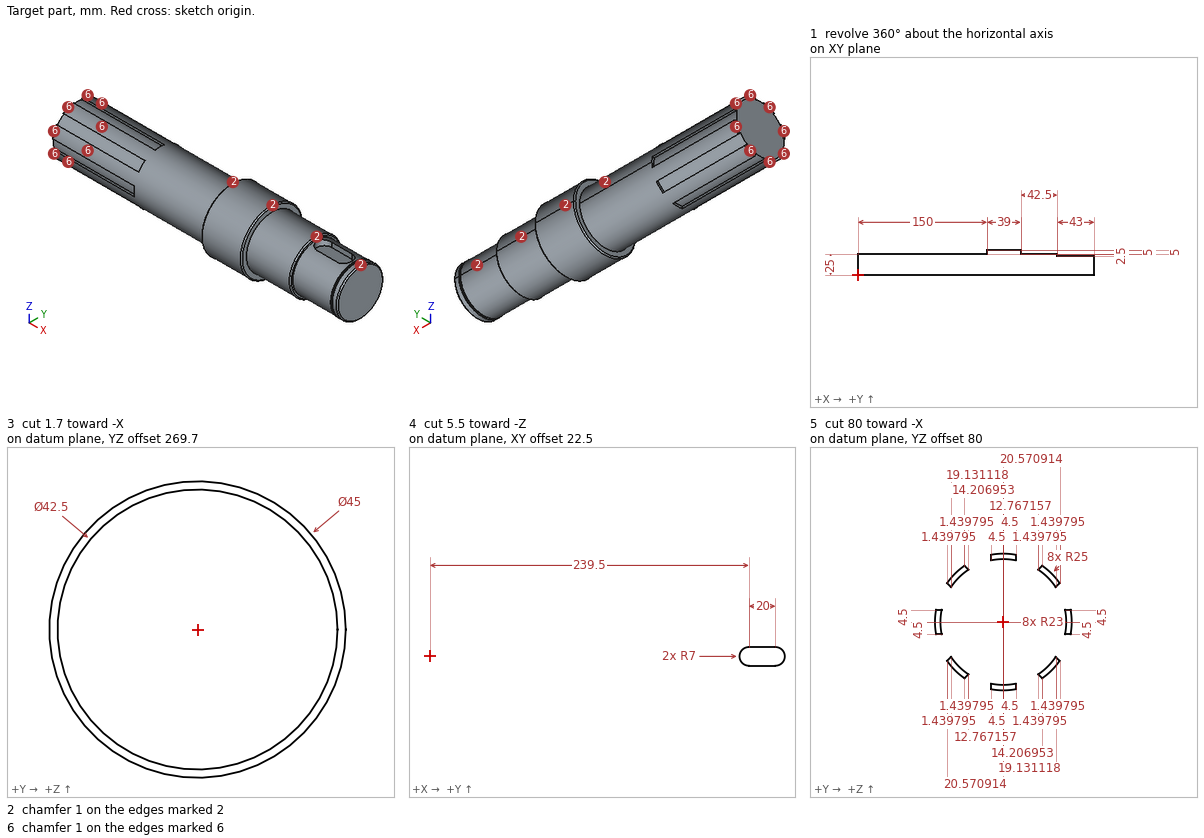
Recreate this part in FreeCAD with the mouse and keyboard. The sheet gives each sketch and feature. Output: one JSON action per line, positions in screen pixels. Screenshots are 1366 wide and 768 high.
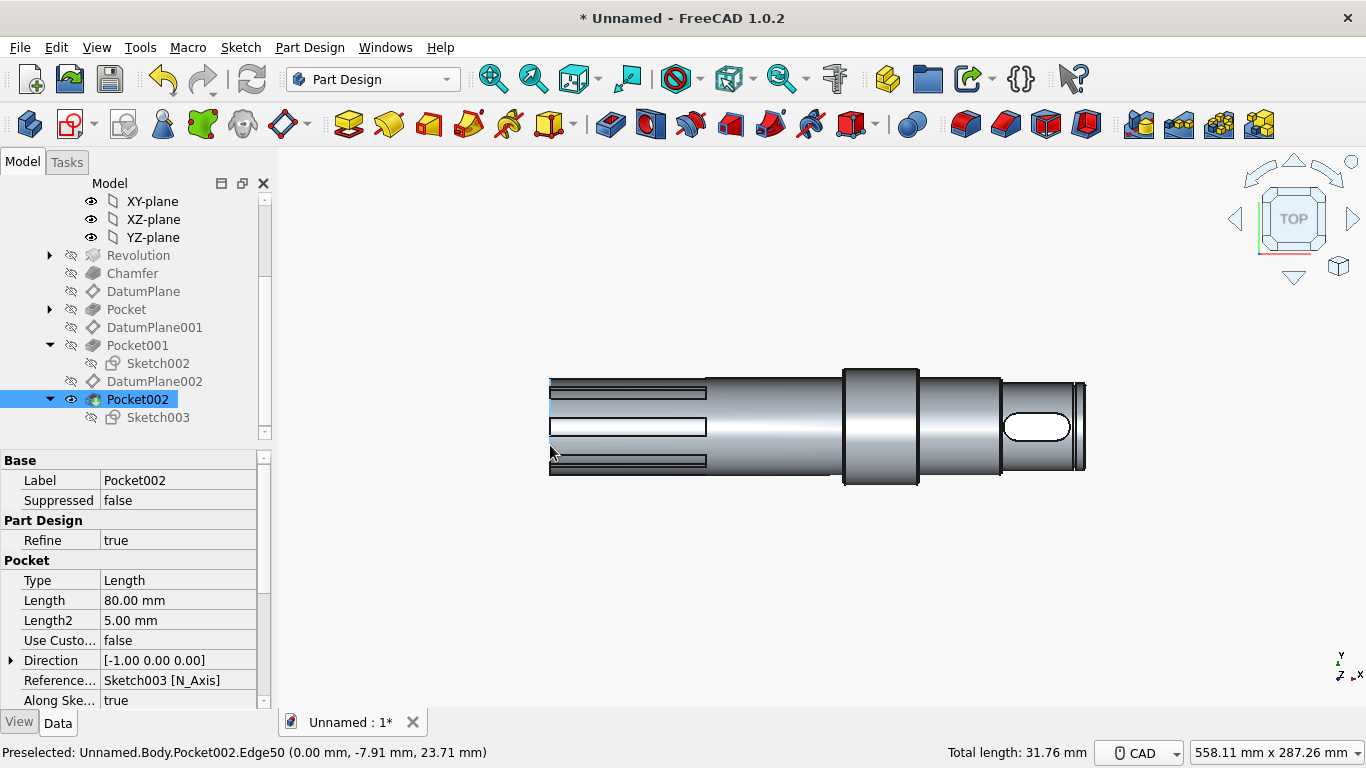
{"action": "left_click", "coordinate": [550, 473], "text": "ctrl"}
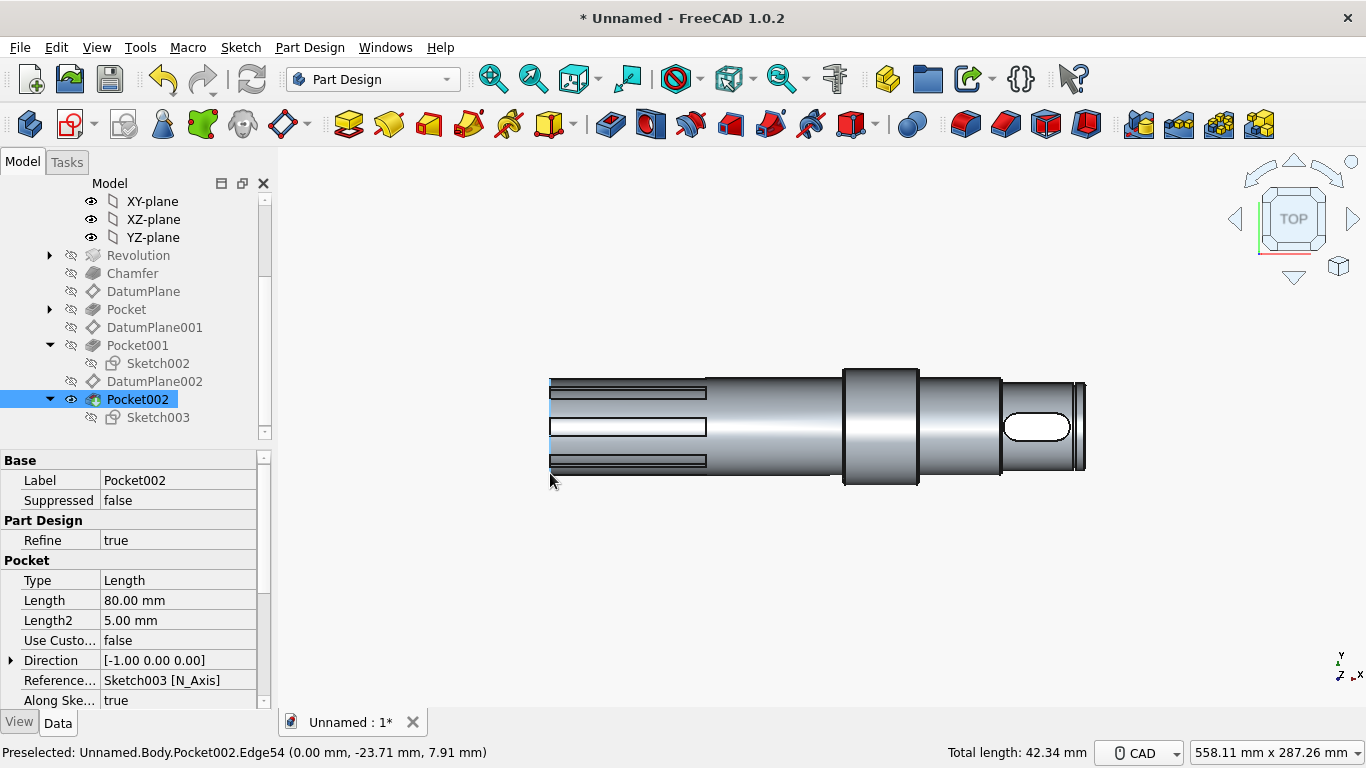
{"action": "scroll", "coordinate": [550, 471], "scroll_direction": "up", "scroll_amount": 4}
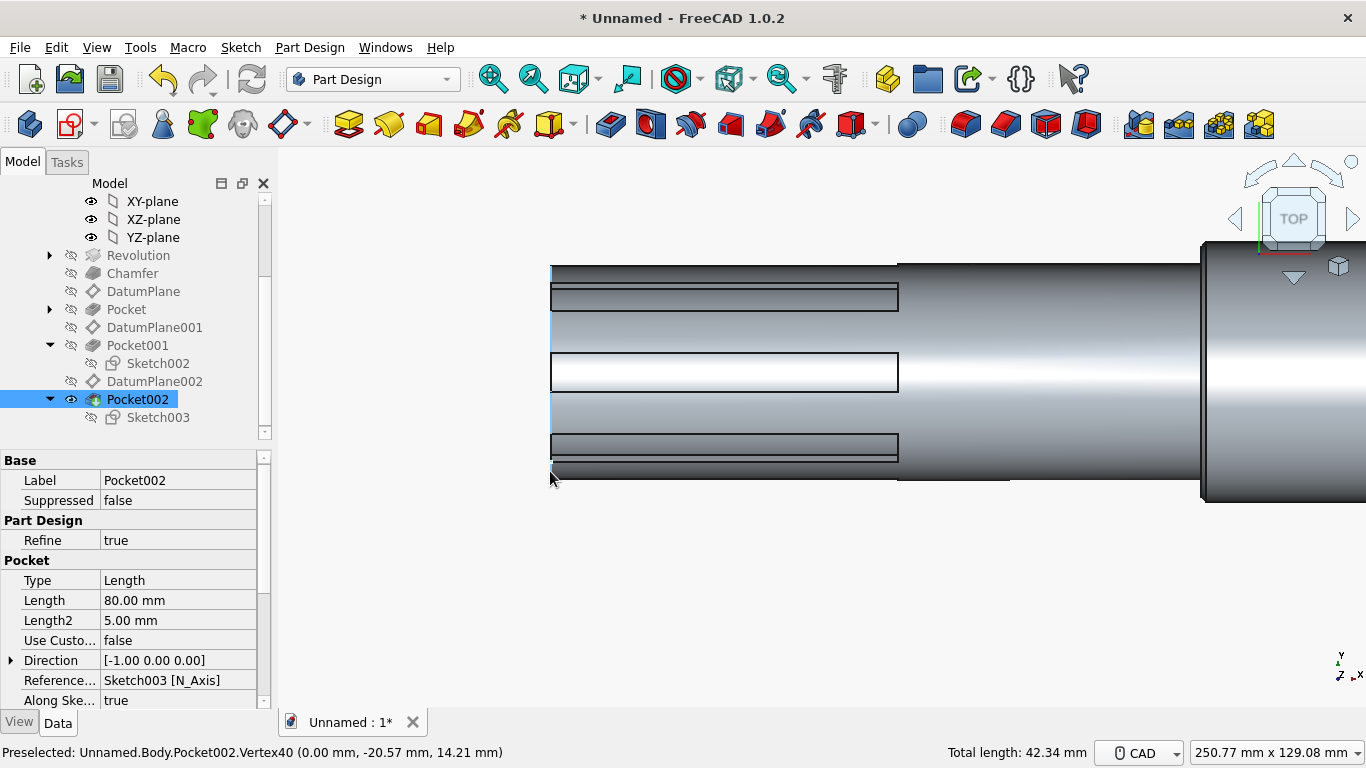
{"action": "key", "text": "v f"}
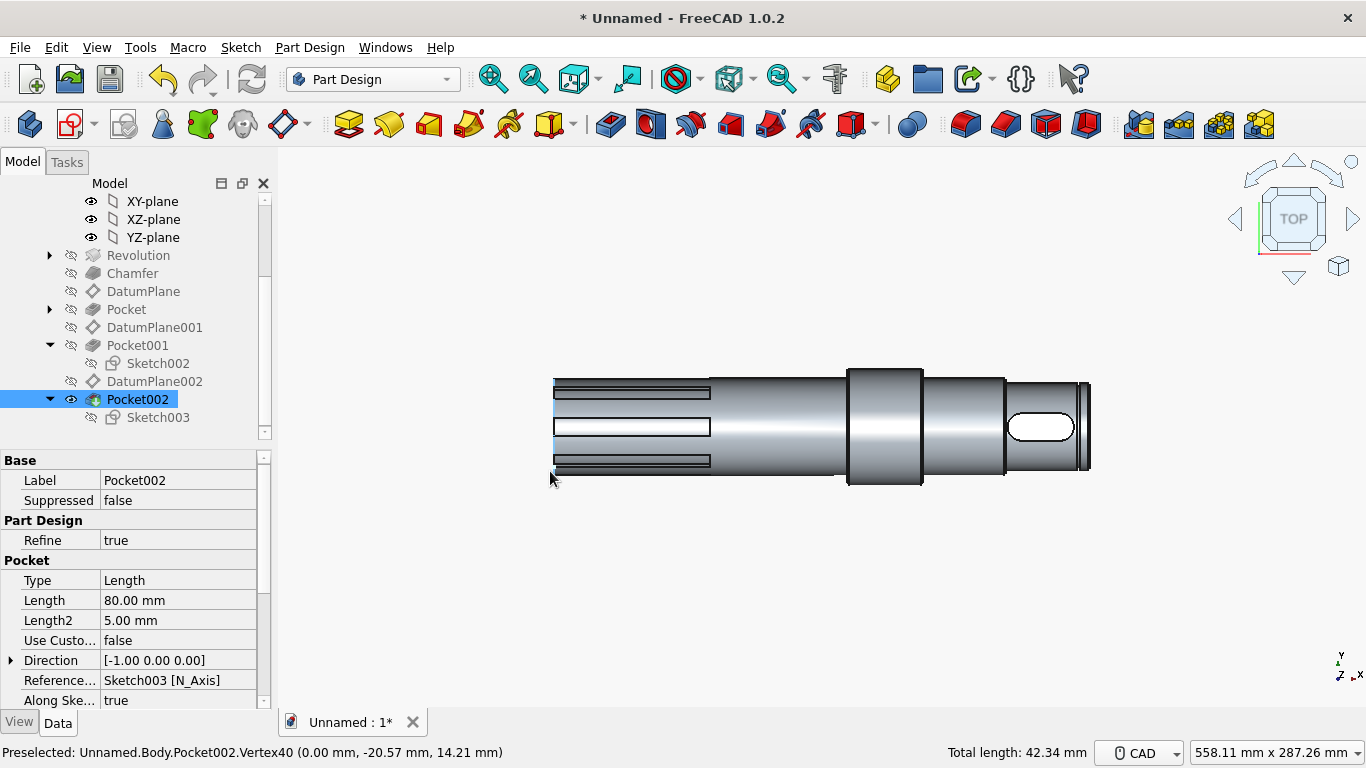
{"action": "key", "text": "0"}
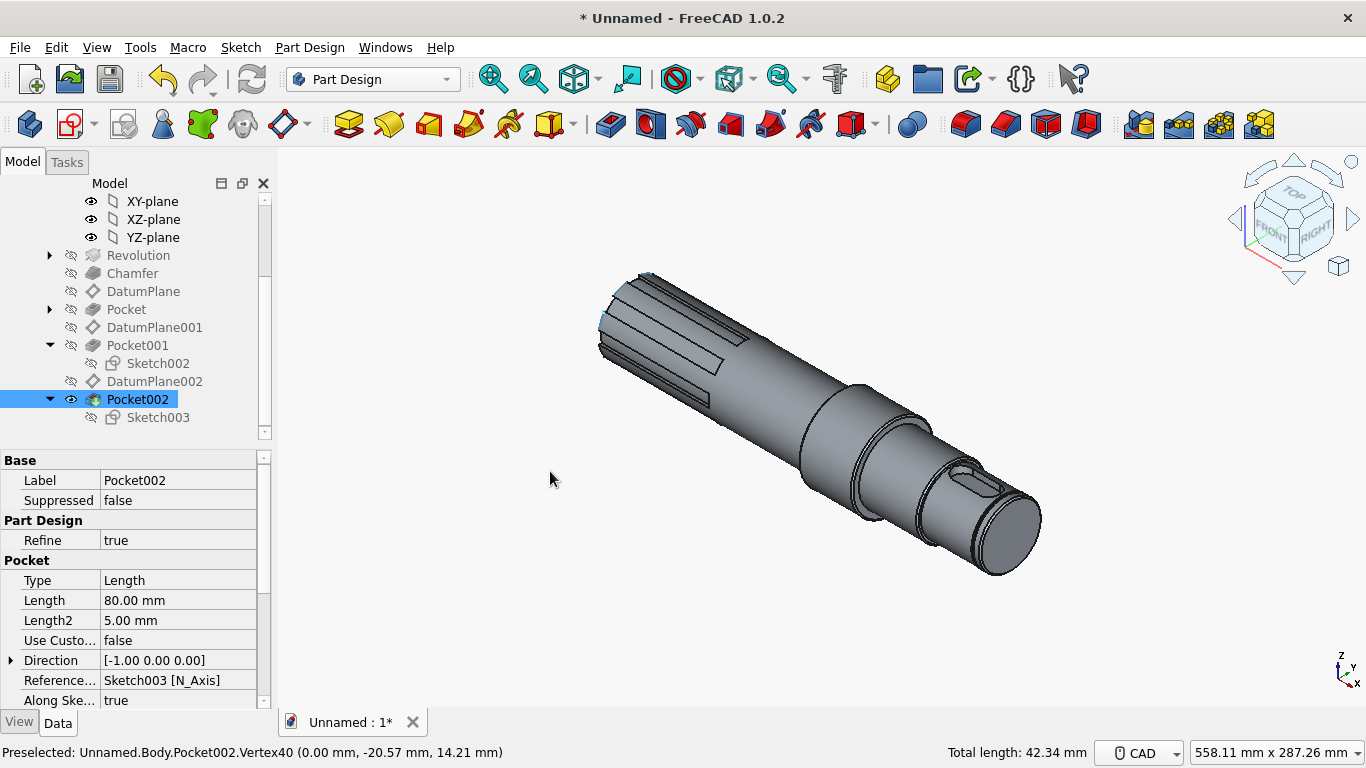
{"action": "left_click", "coordinate": [603, 355], "text": "ctrl"}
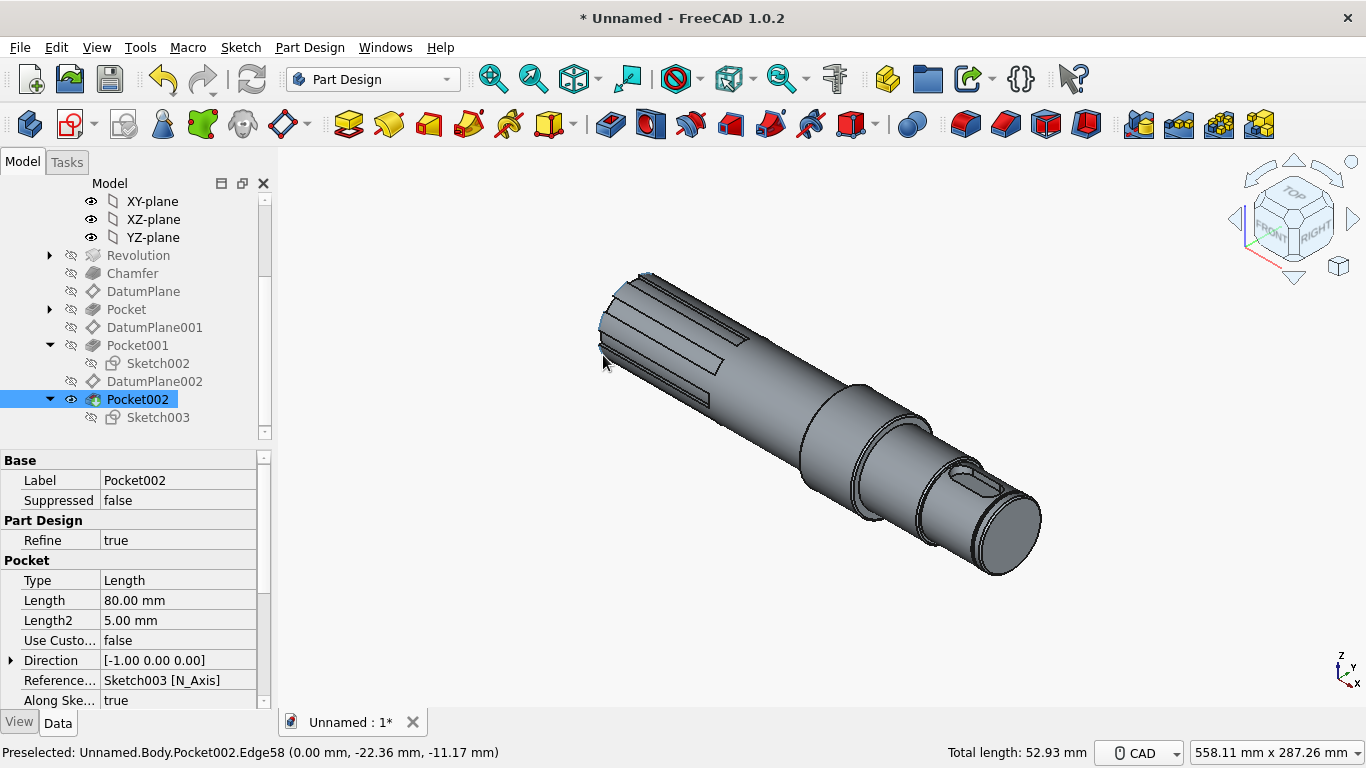
{"action": "scroll", "coordinate": [620, 361], "scroll_direction": "up", "scroll_amount": 4}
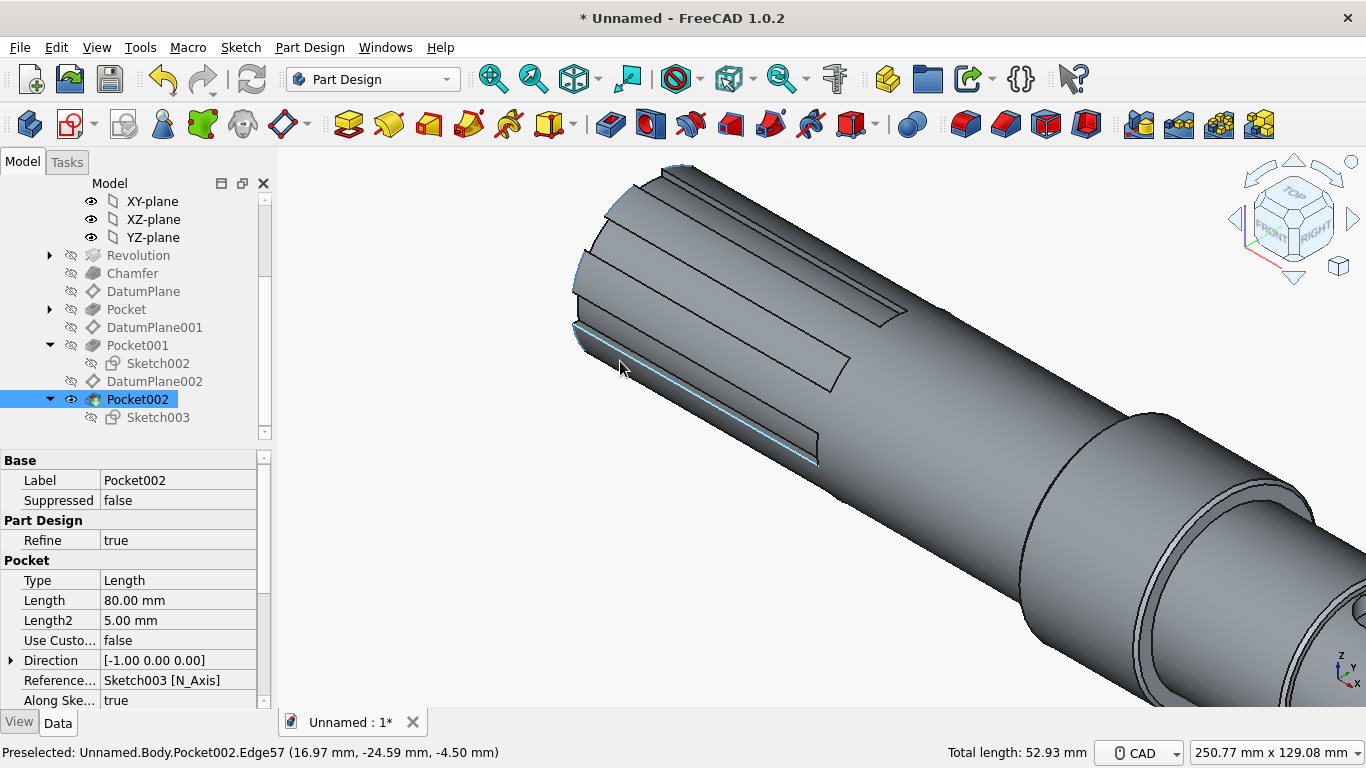
{"action": "left_click", "coordinate": [494, 80]}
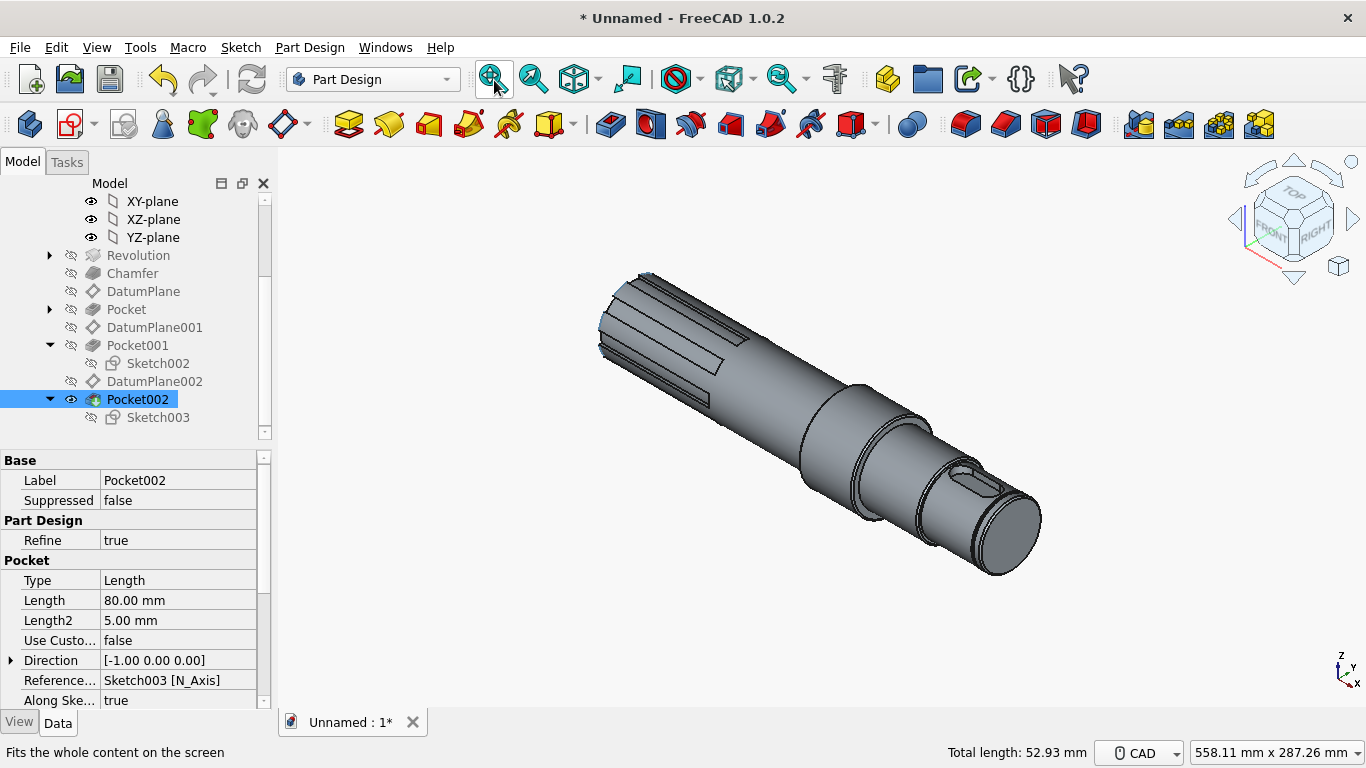
{"action": "key", "text": "2"}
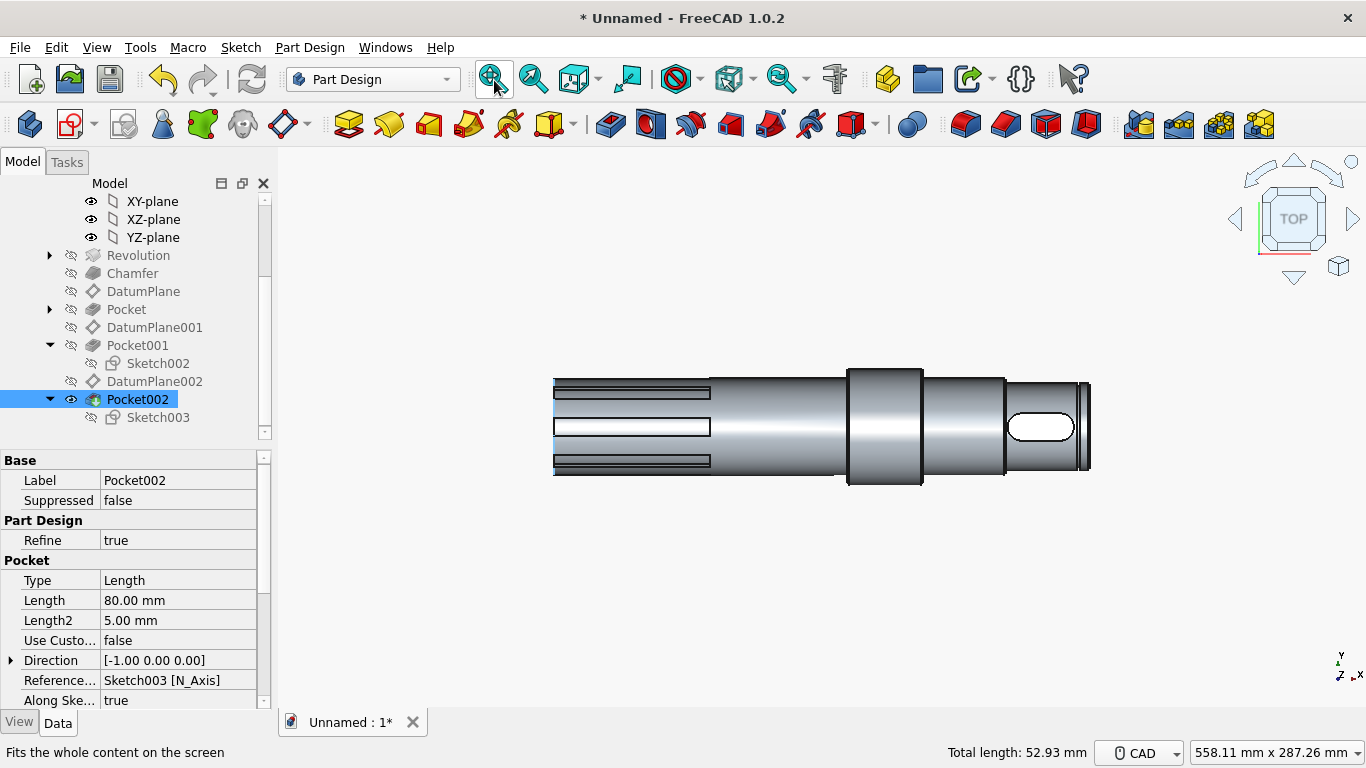
{"action": "scroll", "coordinate": [554, 445], "scroll_direction": "up", "scroll_amount": 4}